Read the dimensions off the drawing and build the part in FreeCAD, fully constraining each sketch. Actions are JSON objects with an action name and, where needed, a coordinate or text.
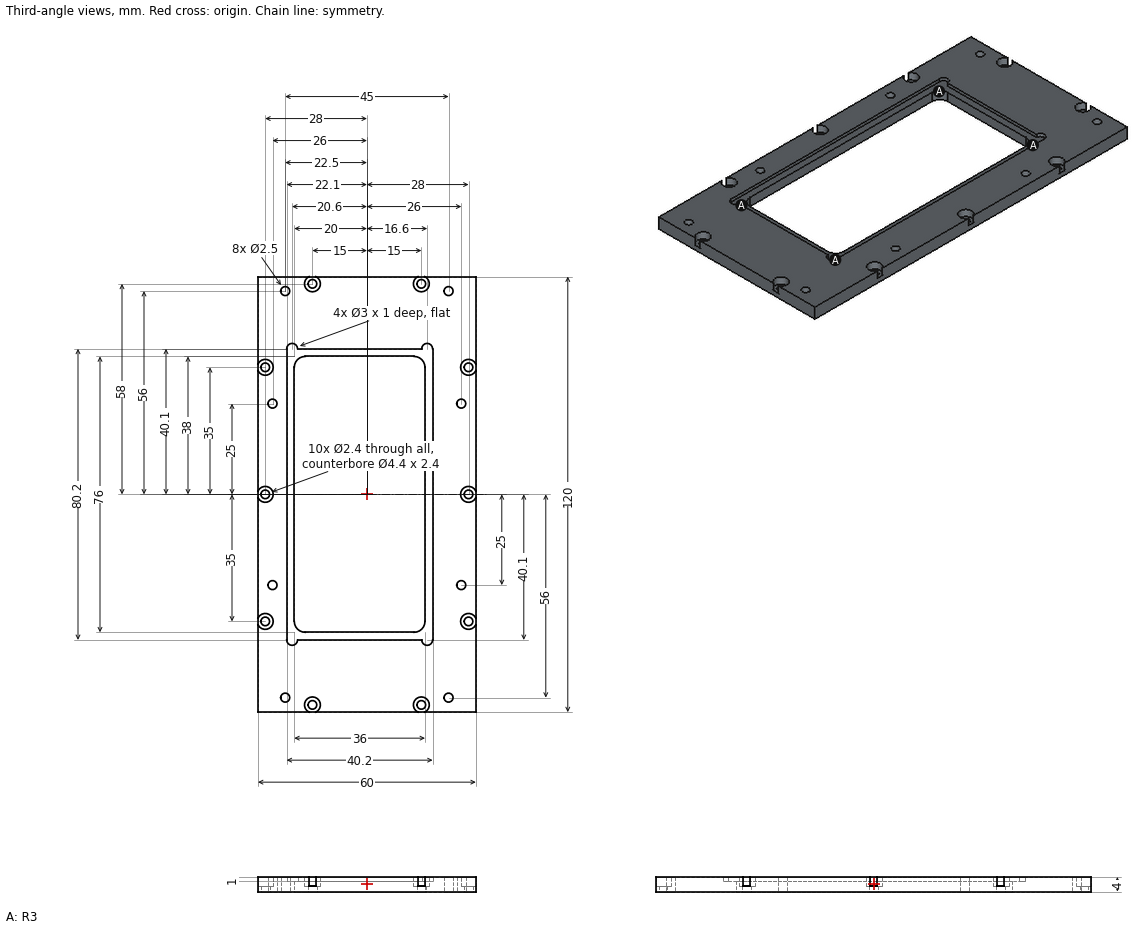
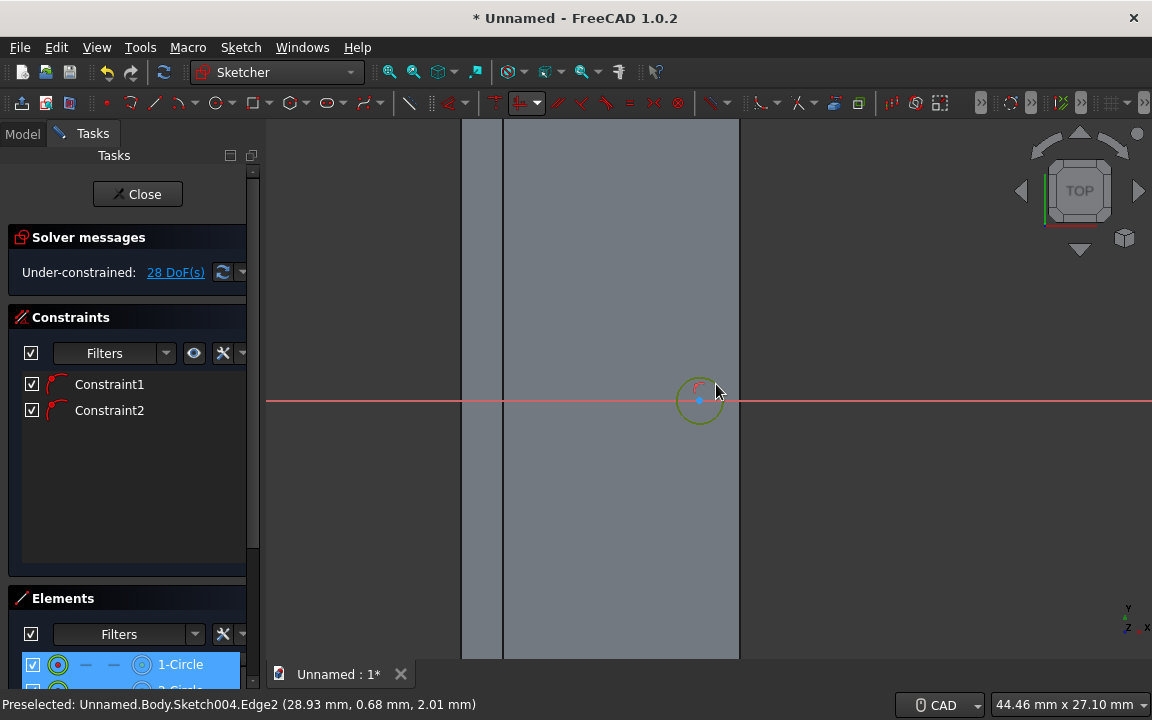
{"action": "scroll", "coordinate": [718, 387], "scroll_direction": "down", "scroll_amount": 10}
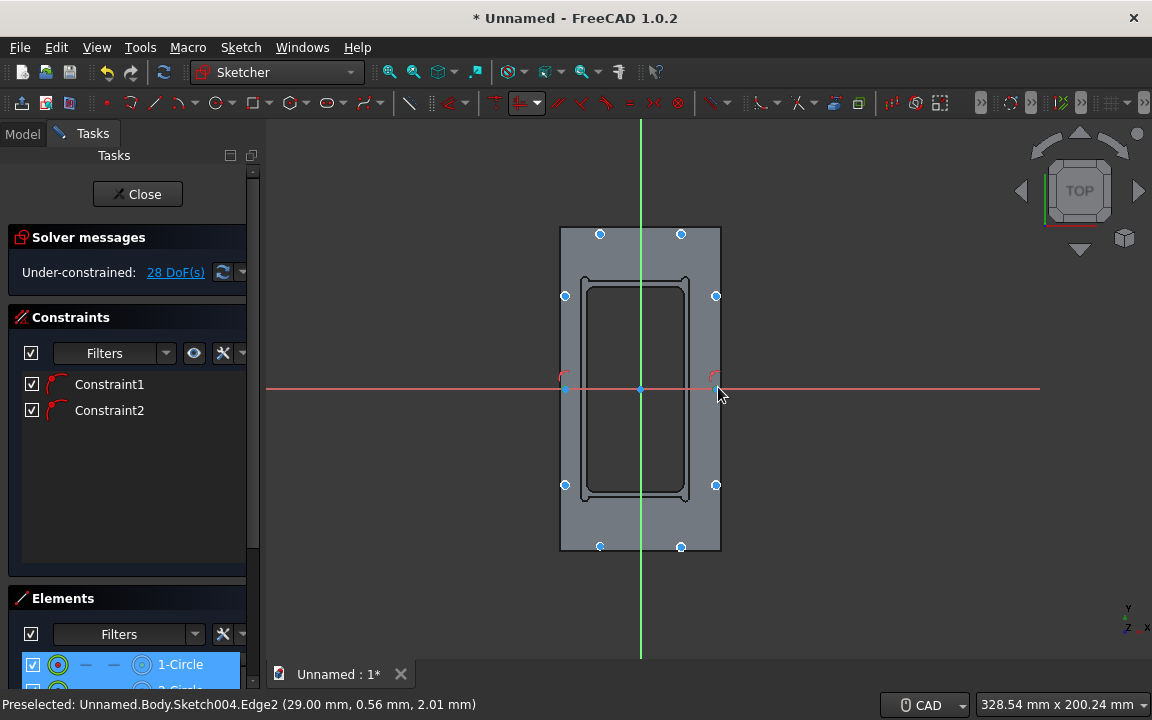
{"action": "scroll", "coordinate": [603, 231], "scroll_direction": "up", "scroll_amount": 7}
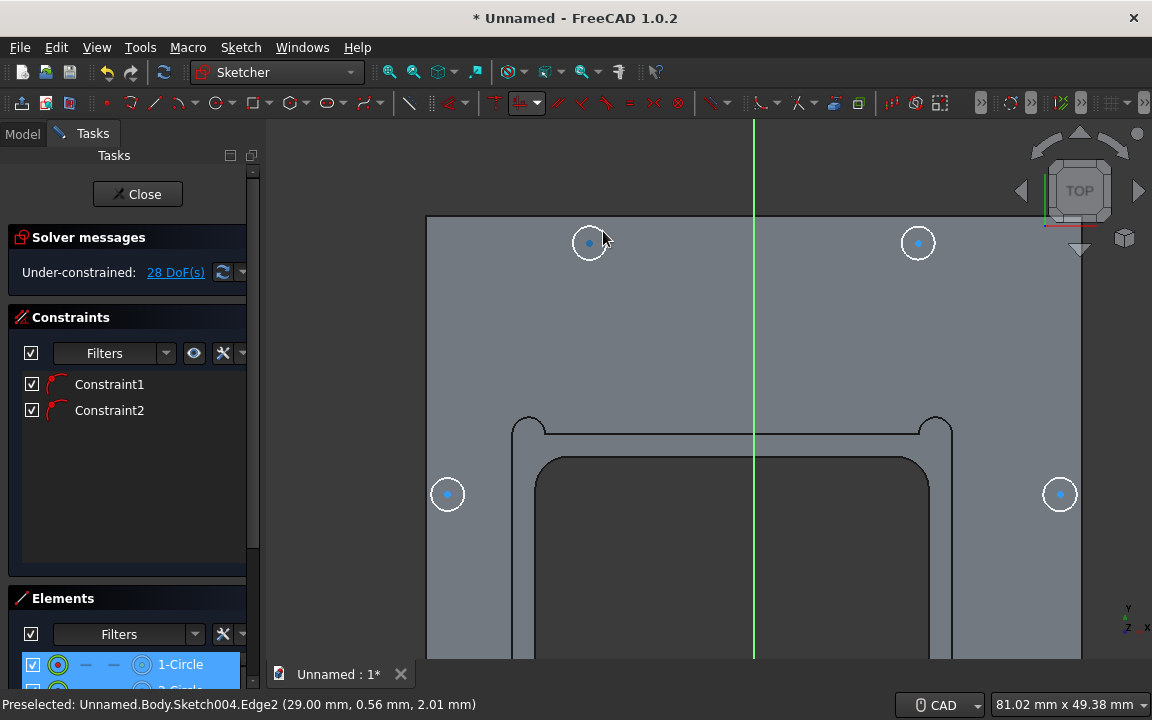
{"action": "left_click", "coordinate": [601, 231]}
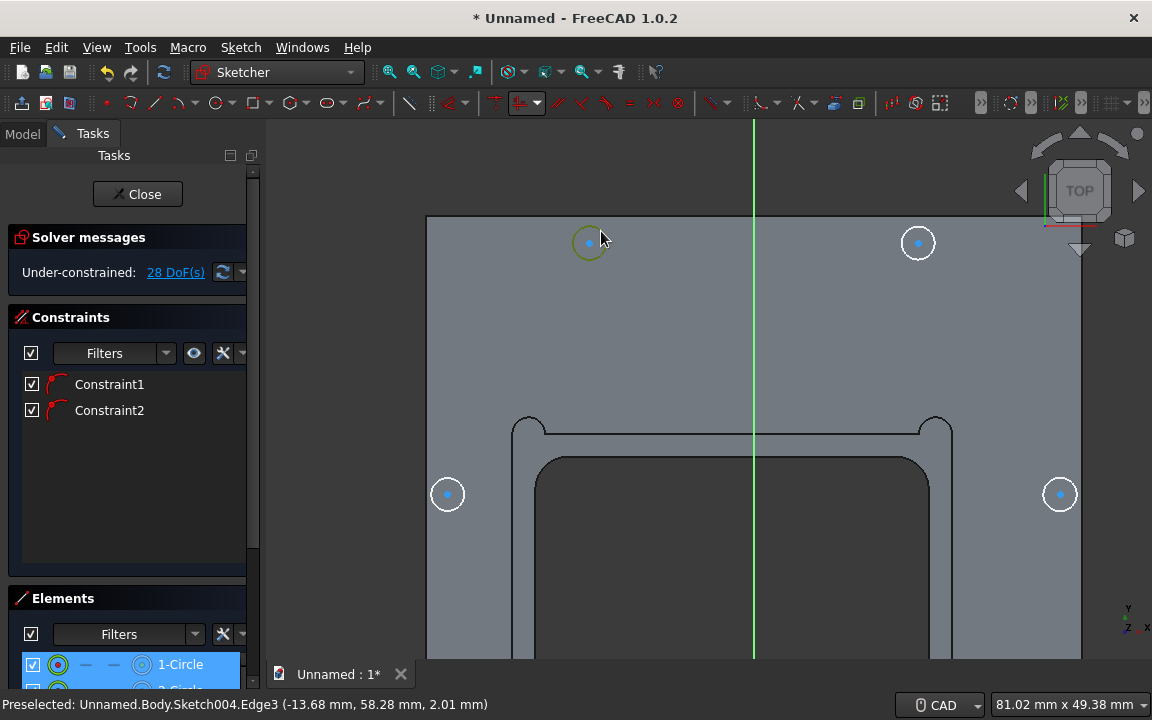
{"action": "left_click", "coordinate": [930, 231]}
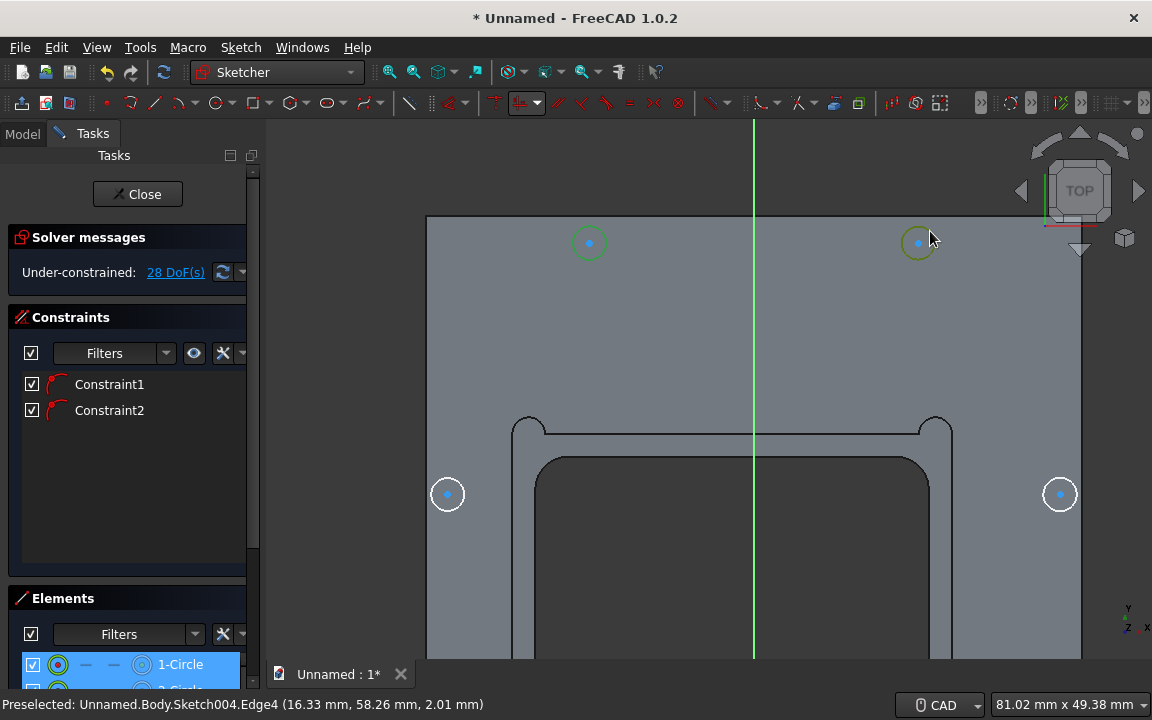
{"action": "left_click", "coordinate": [459, 483]}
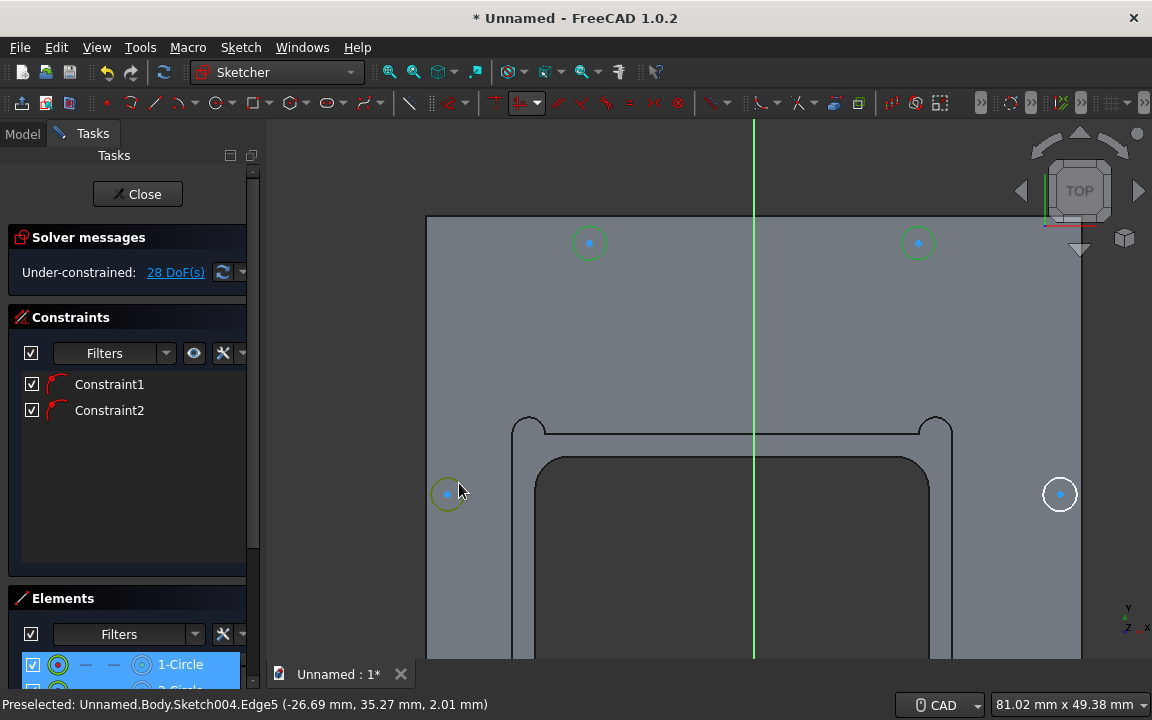
{"action": "scroll", "coordinate": [603, 231], "scroll_direction": "down", "scroll_amount": 7}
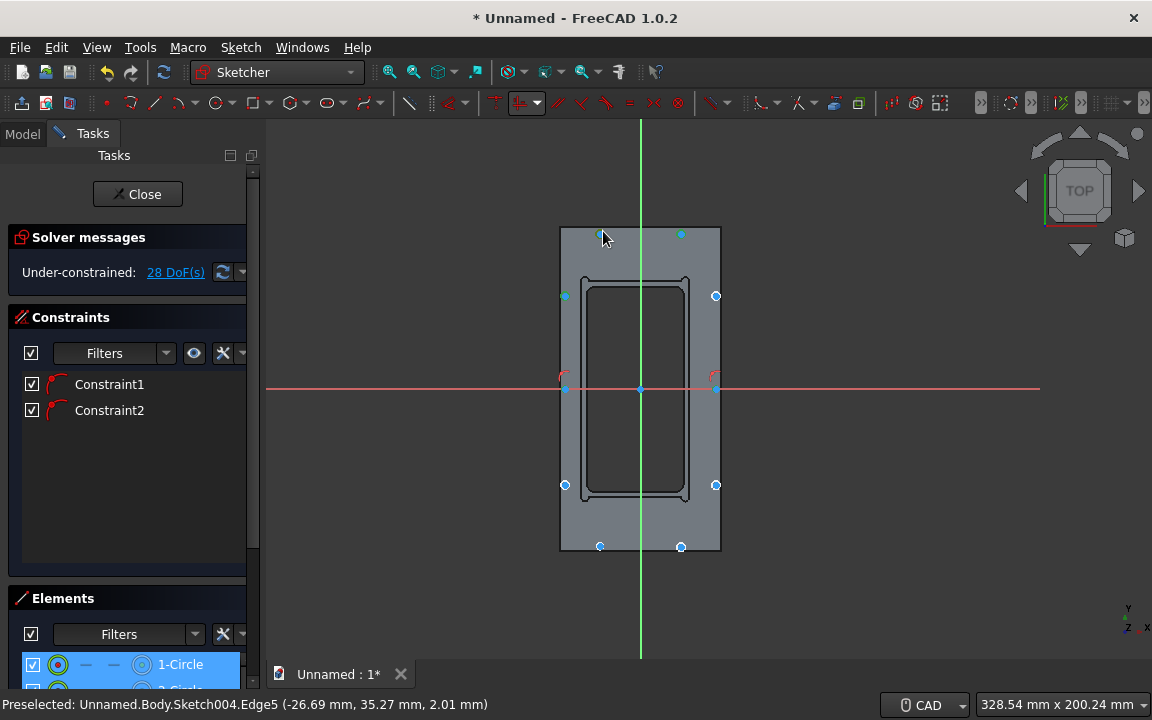
{"action": "scroll", "coordinate": [719, 293], "scroll_direction": "up", "scroll_amount": 7}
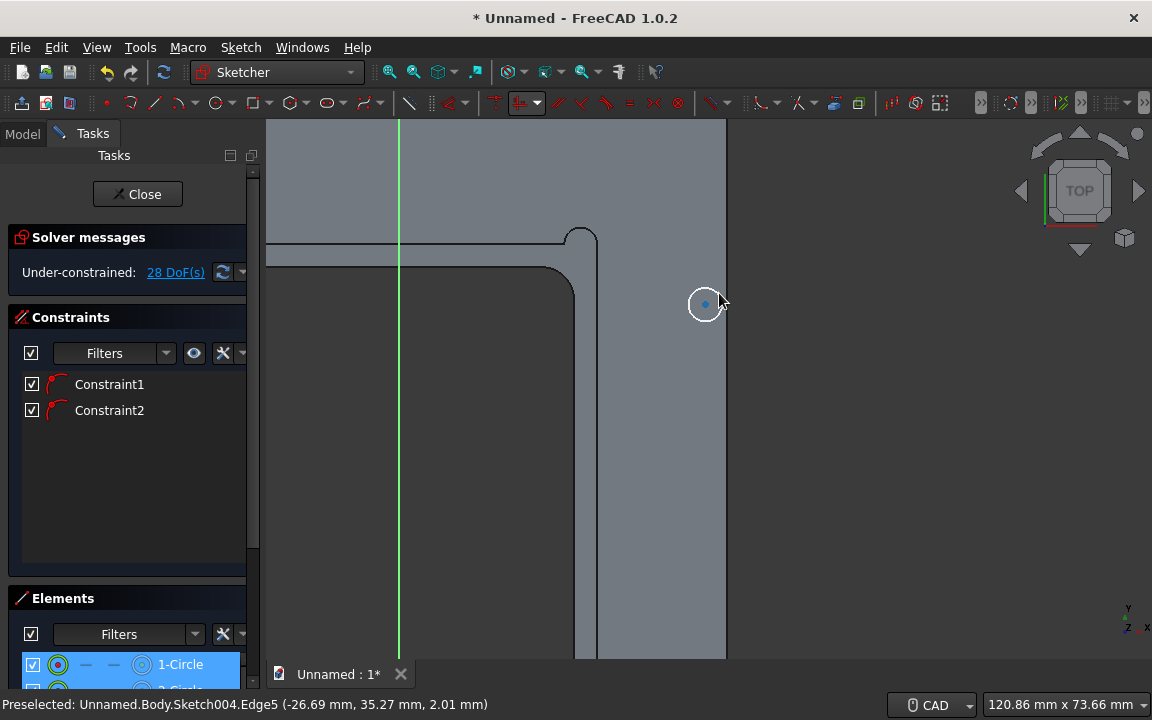
{"action": "left_click", "coordinate": [717, 293]}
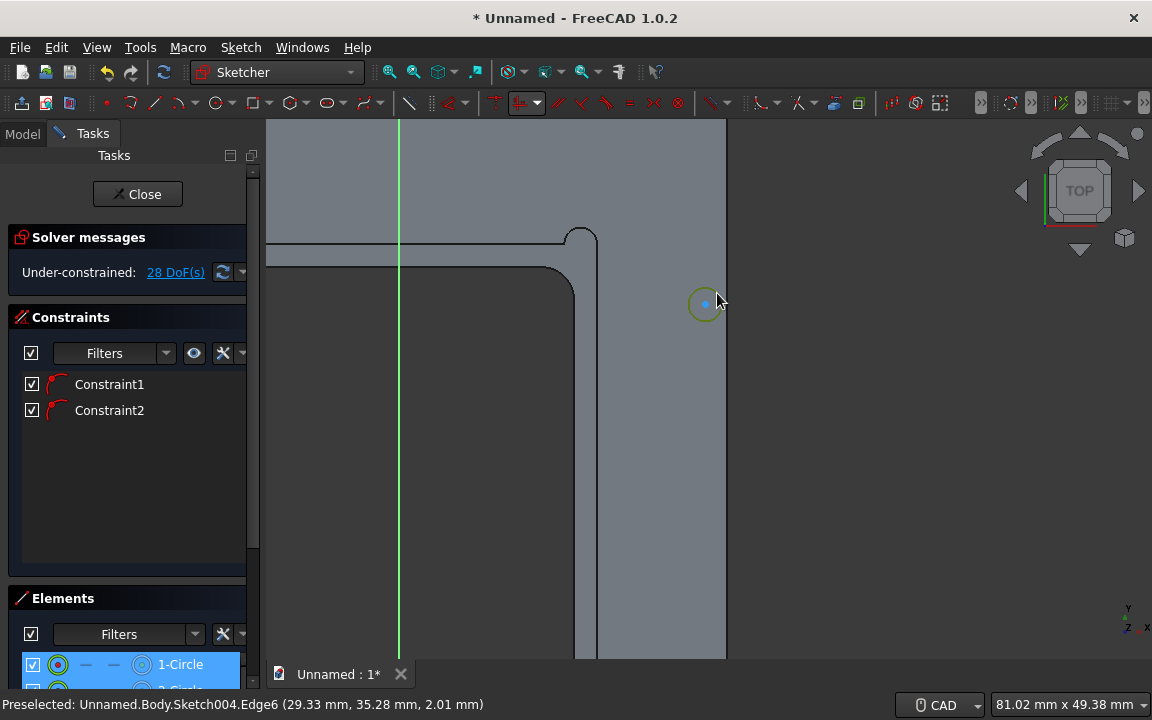
{"action": "scroll", "coordinate": [719, 293], "scroll_direction": "down", "scroll_amount": 7}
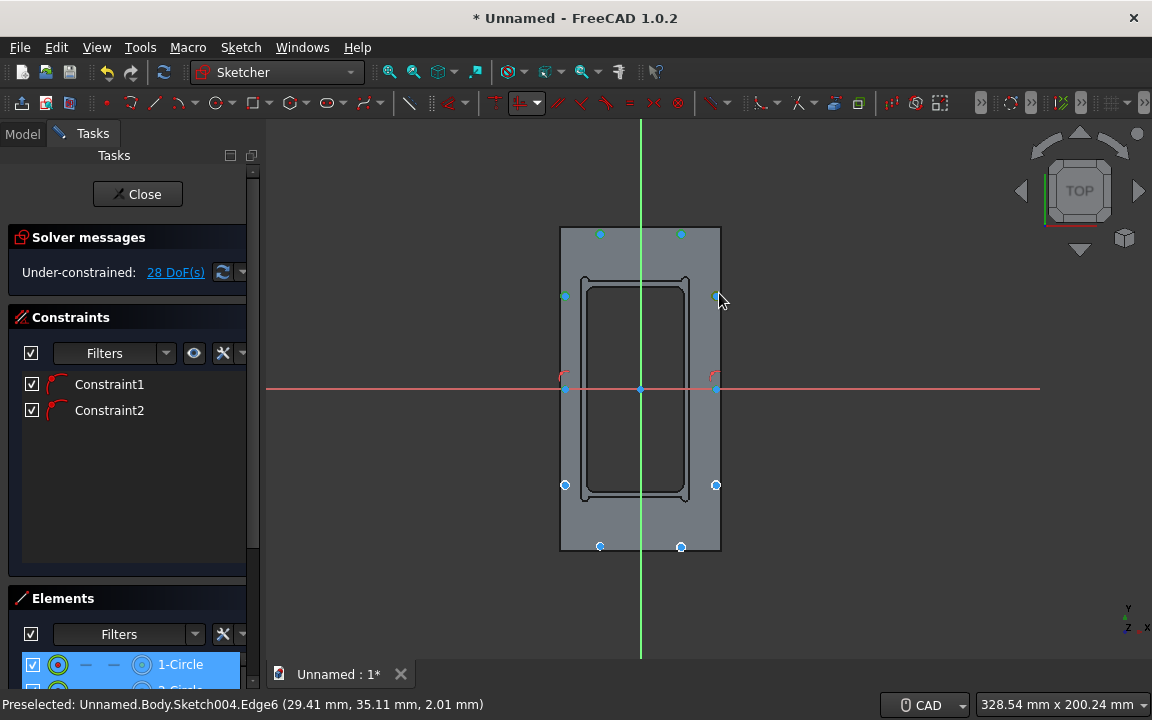
{"action": "scroll", "coordinate": [568, 482], "scroll_direction": "up", "scroll_amount": 7}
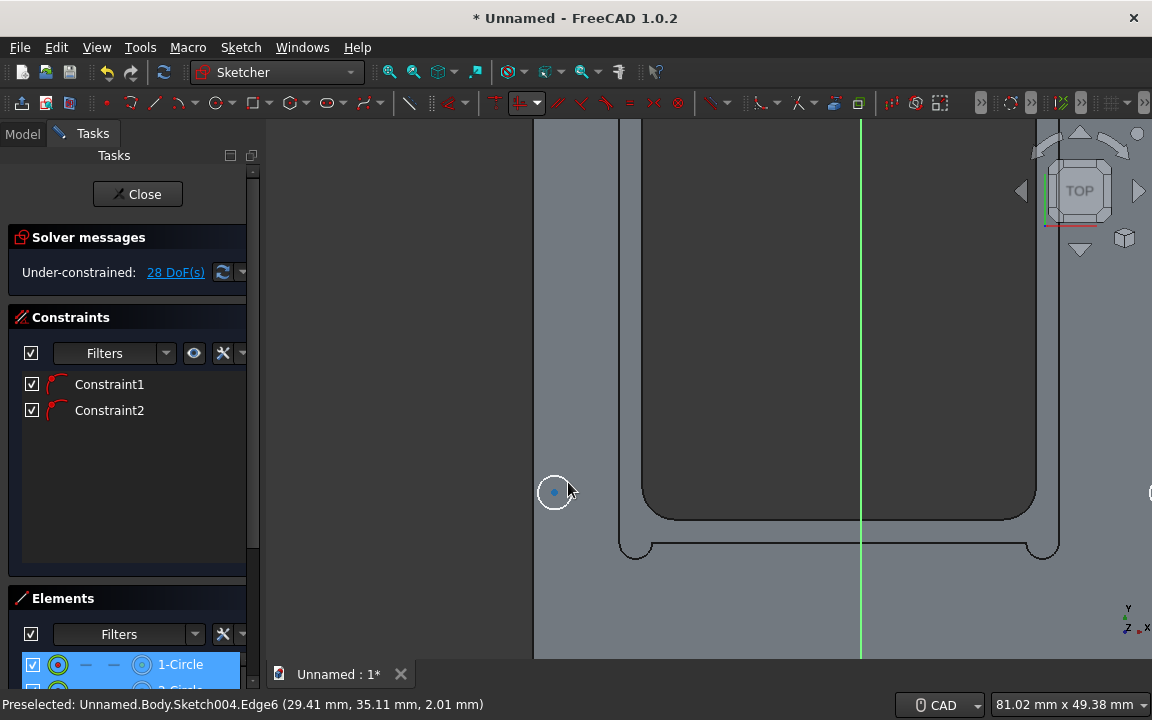
{"action": "left_click", "coordinate": [567, 481]}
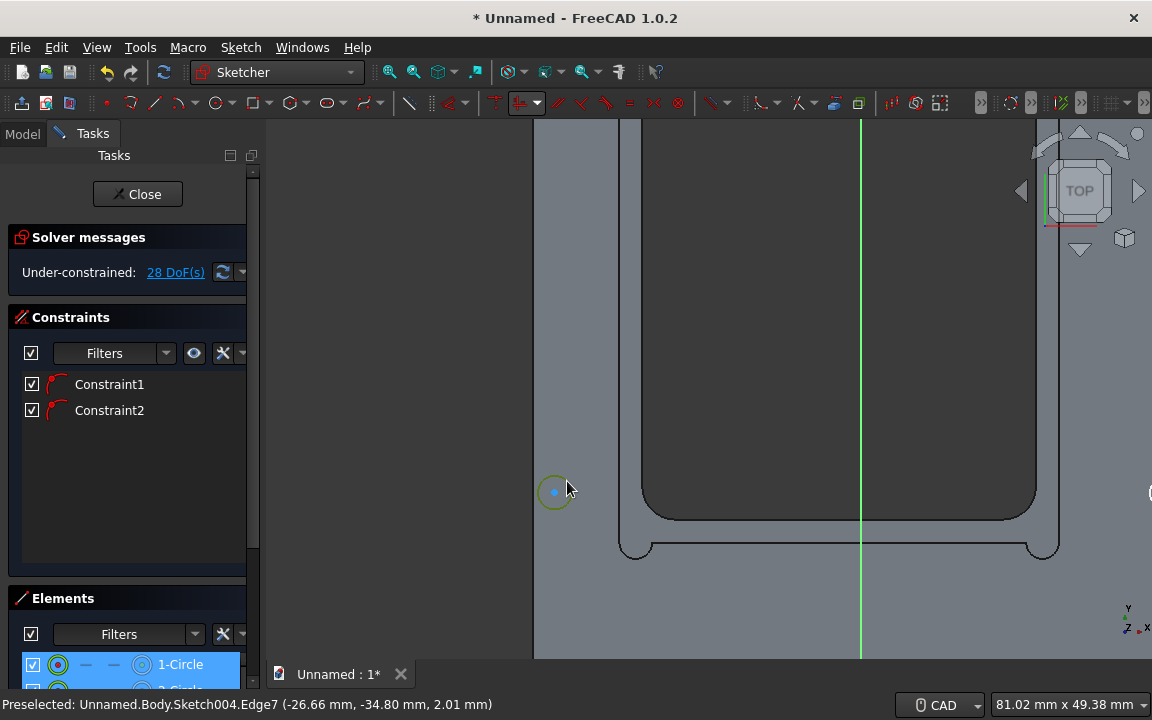
{"action": "scroll", "coordinate": [568, 482], "scroll_direction": "down", "scroll_amount": 7}